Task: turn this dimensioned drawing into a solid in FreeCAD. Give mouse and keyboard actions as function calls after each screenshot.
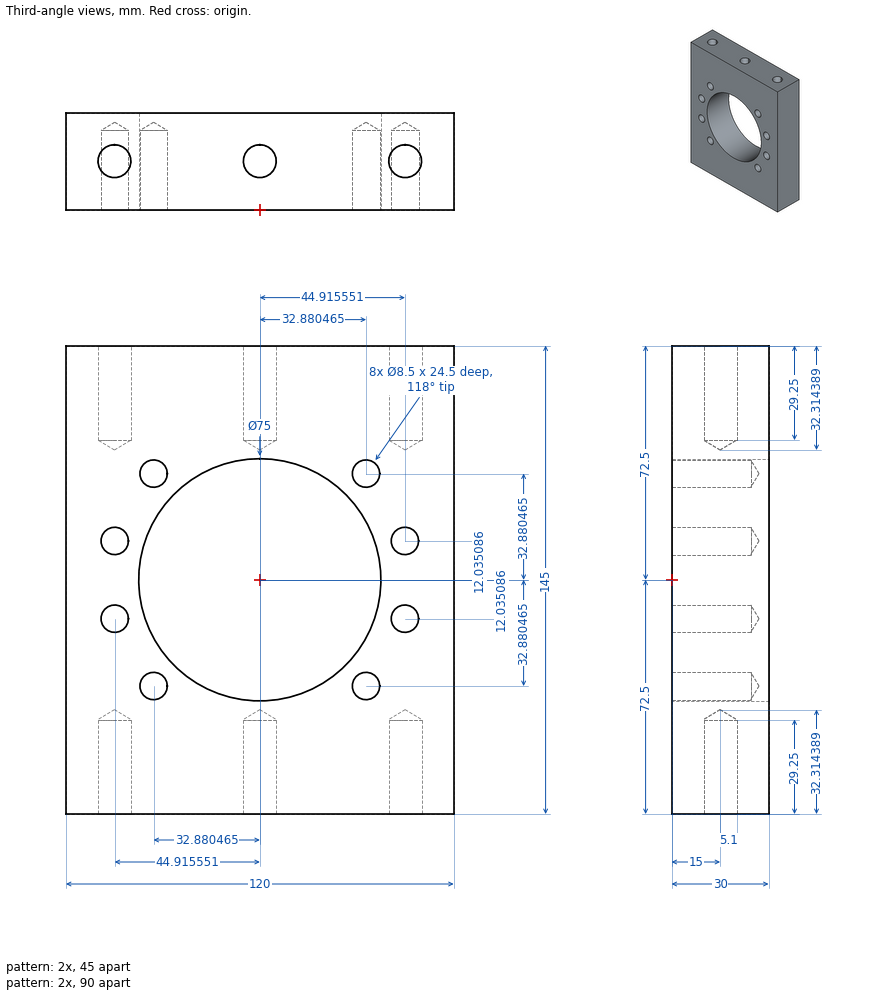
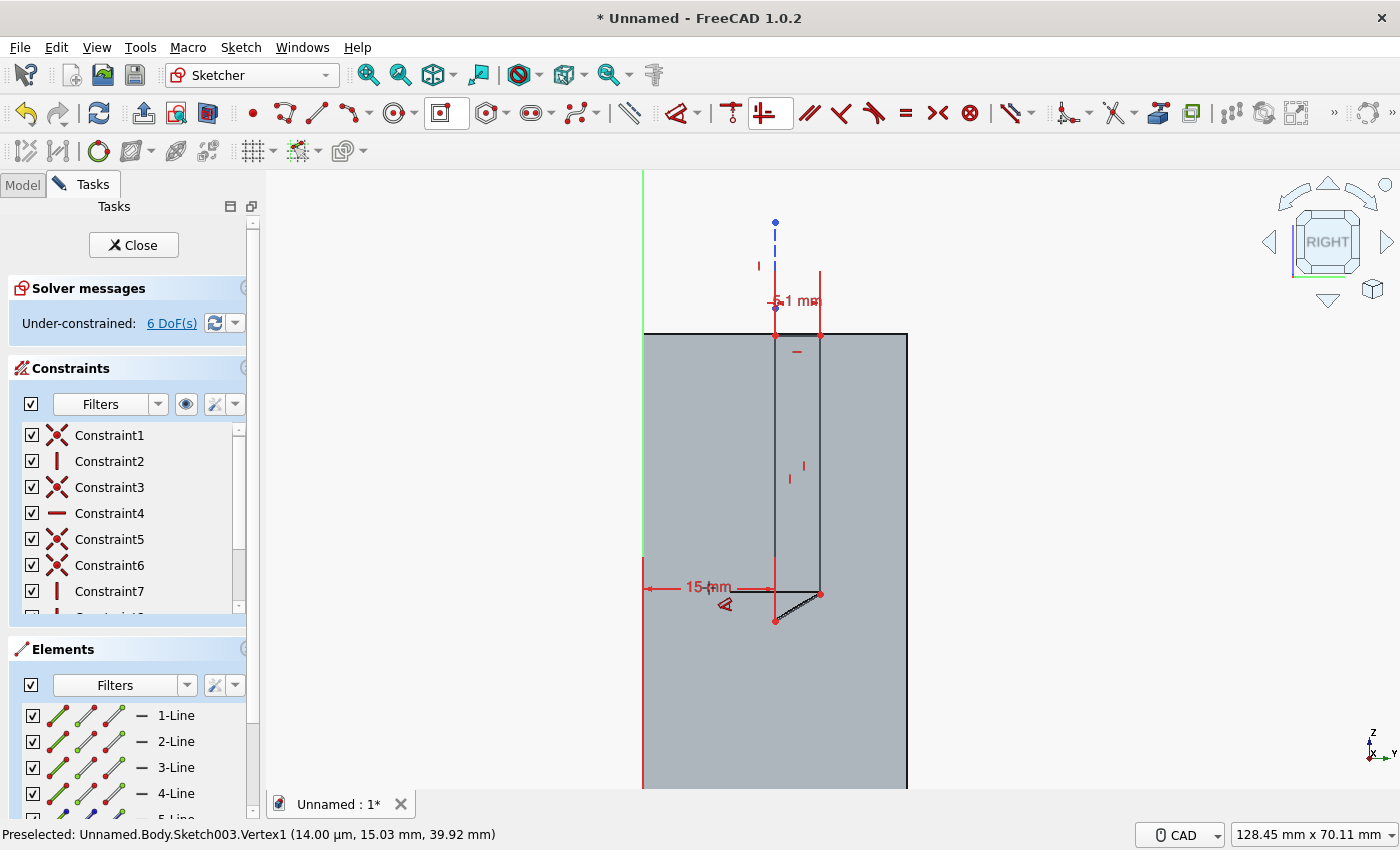
click(775, 308)
click(709, 274)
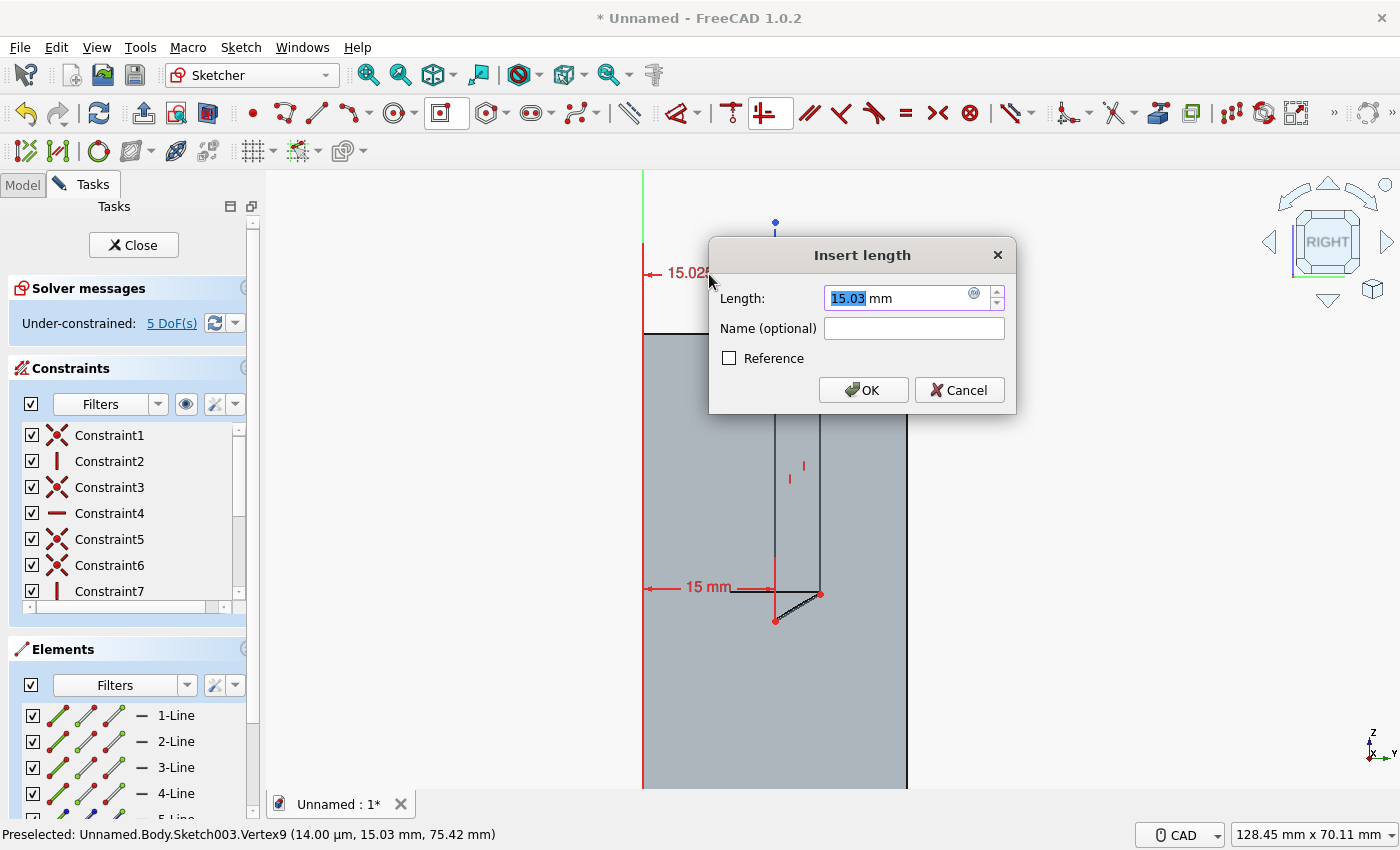
text(15)
key(Return)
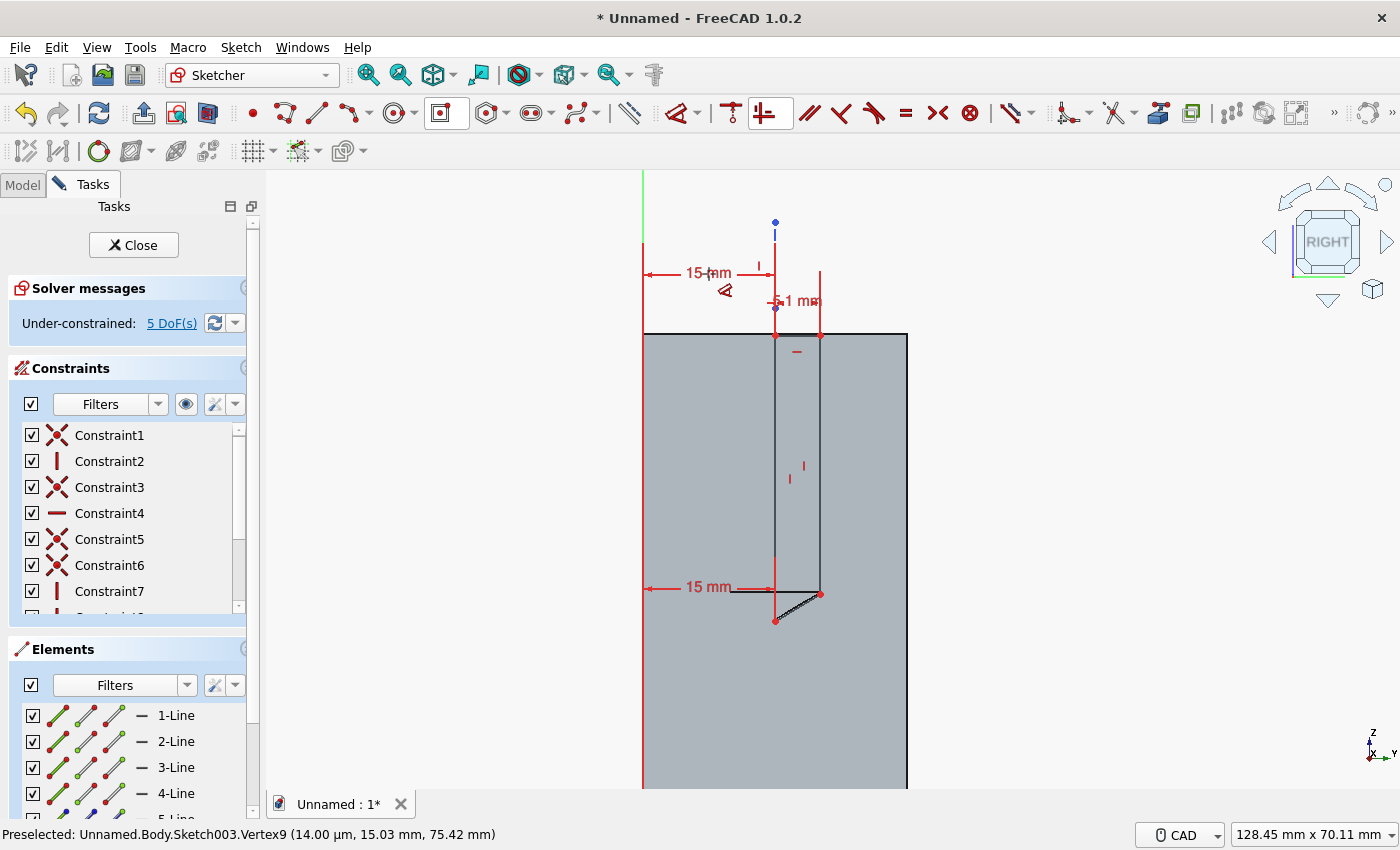
click(820, 517)
click(854, 465)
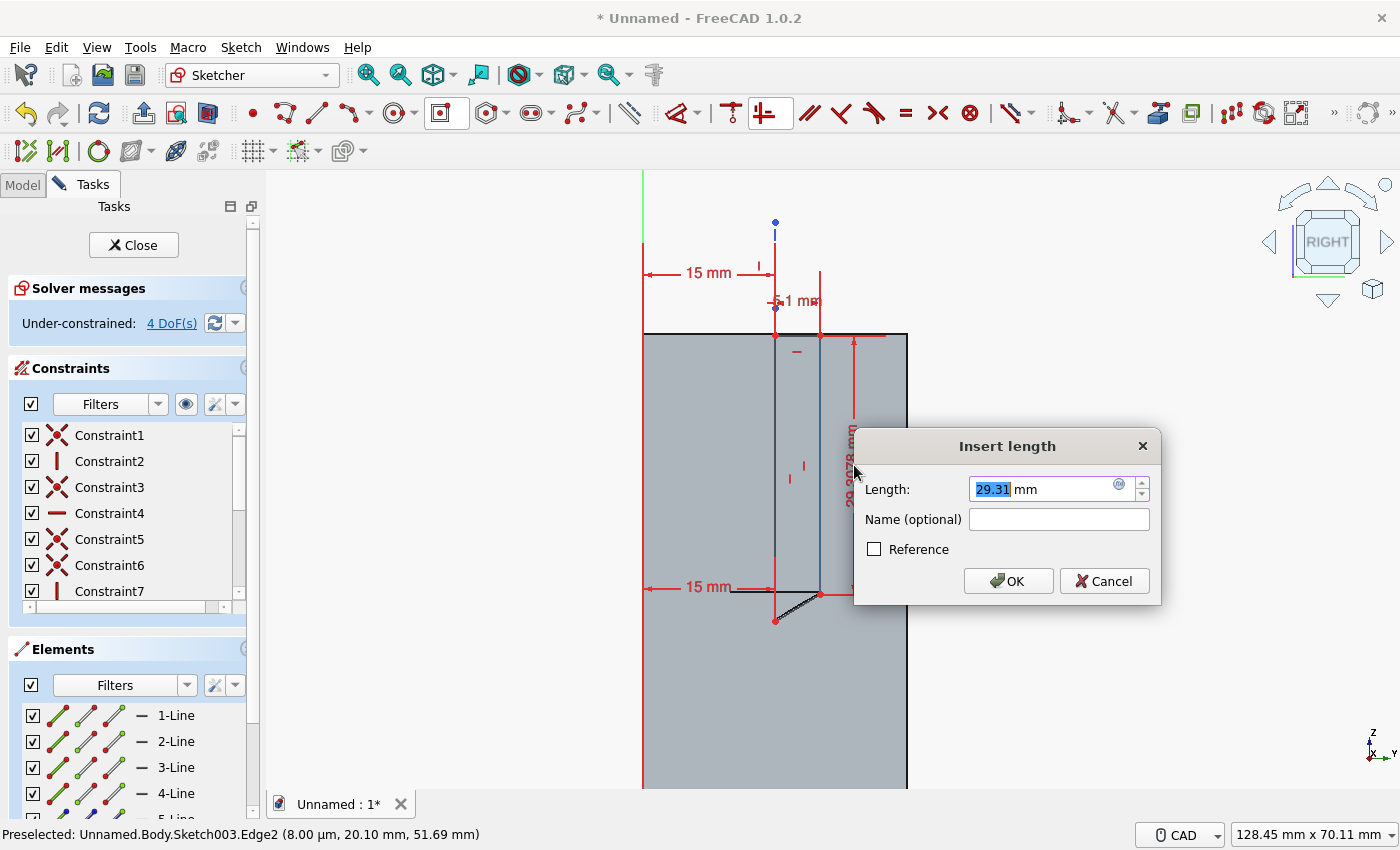
text(29.25)
key(Return)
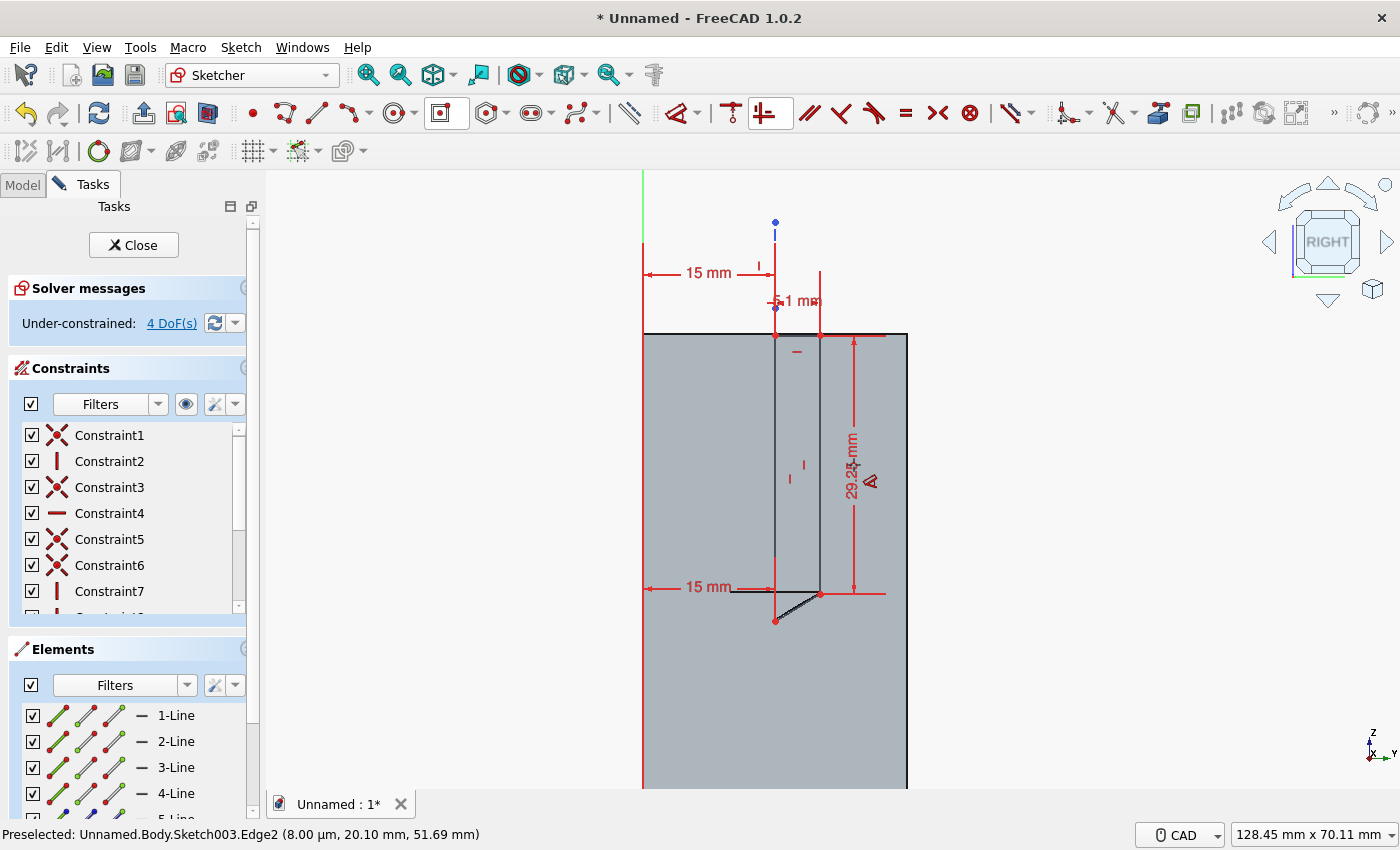
click(820, 336)
click(854, 548)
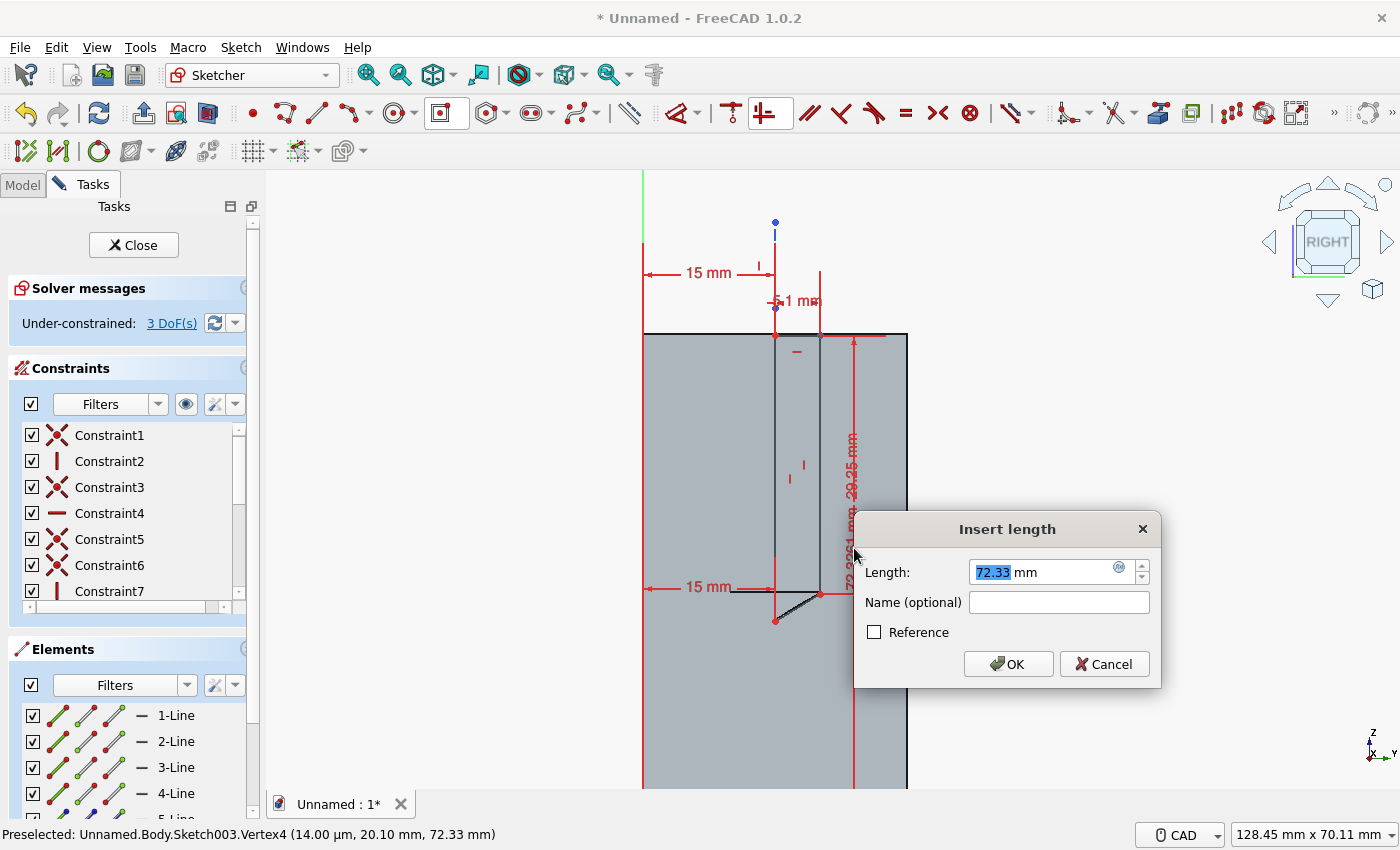
text(72.5)
key(Return)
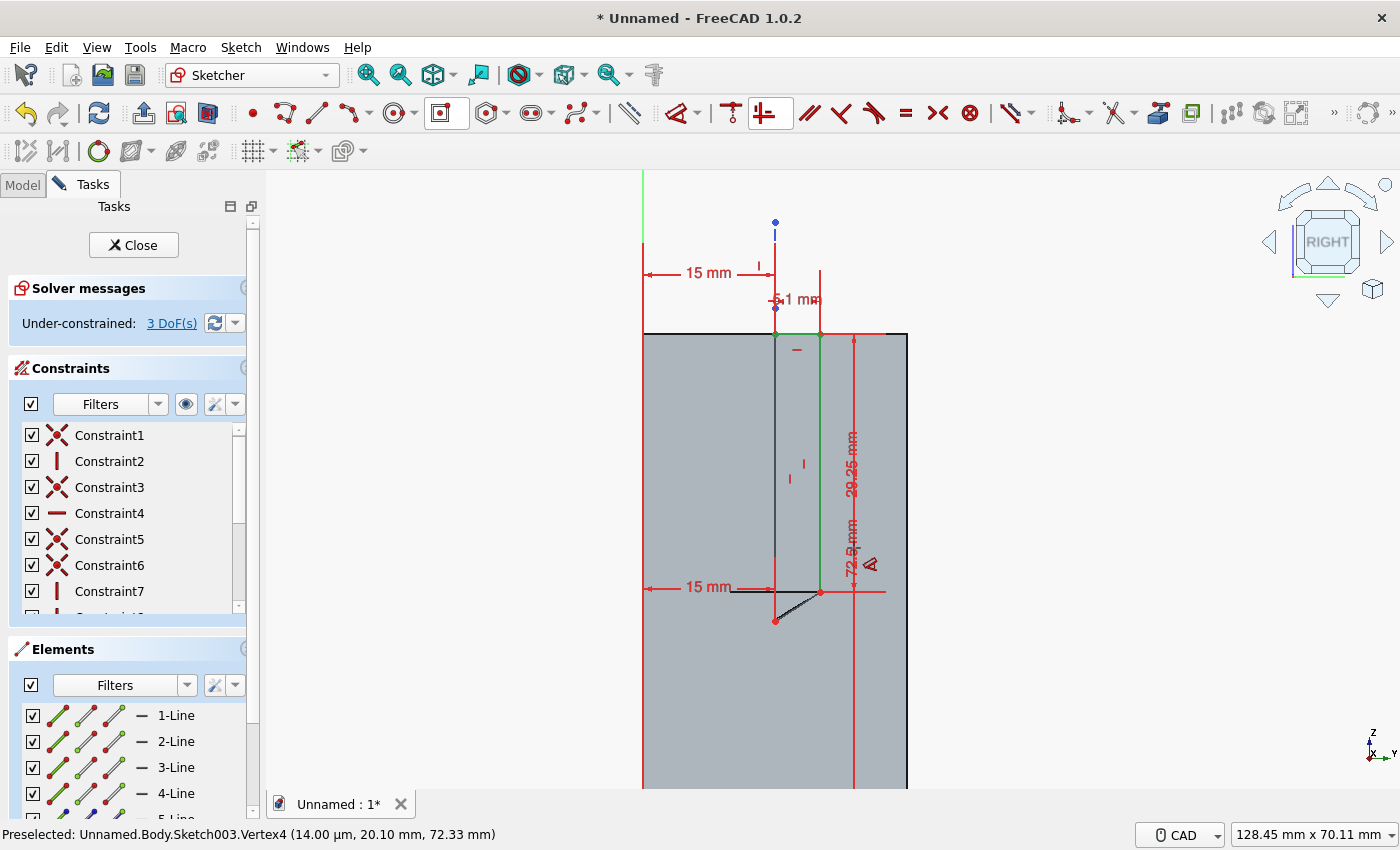
click(775, 421)
click(741, 478)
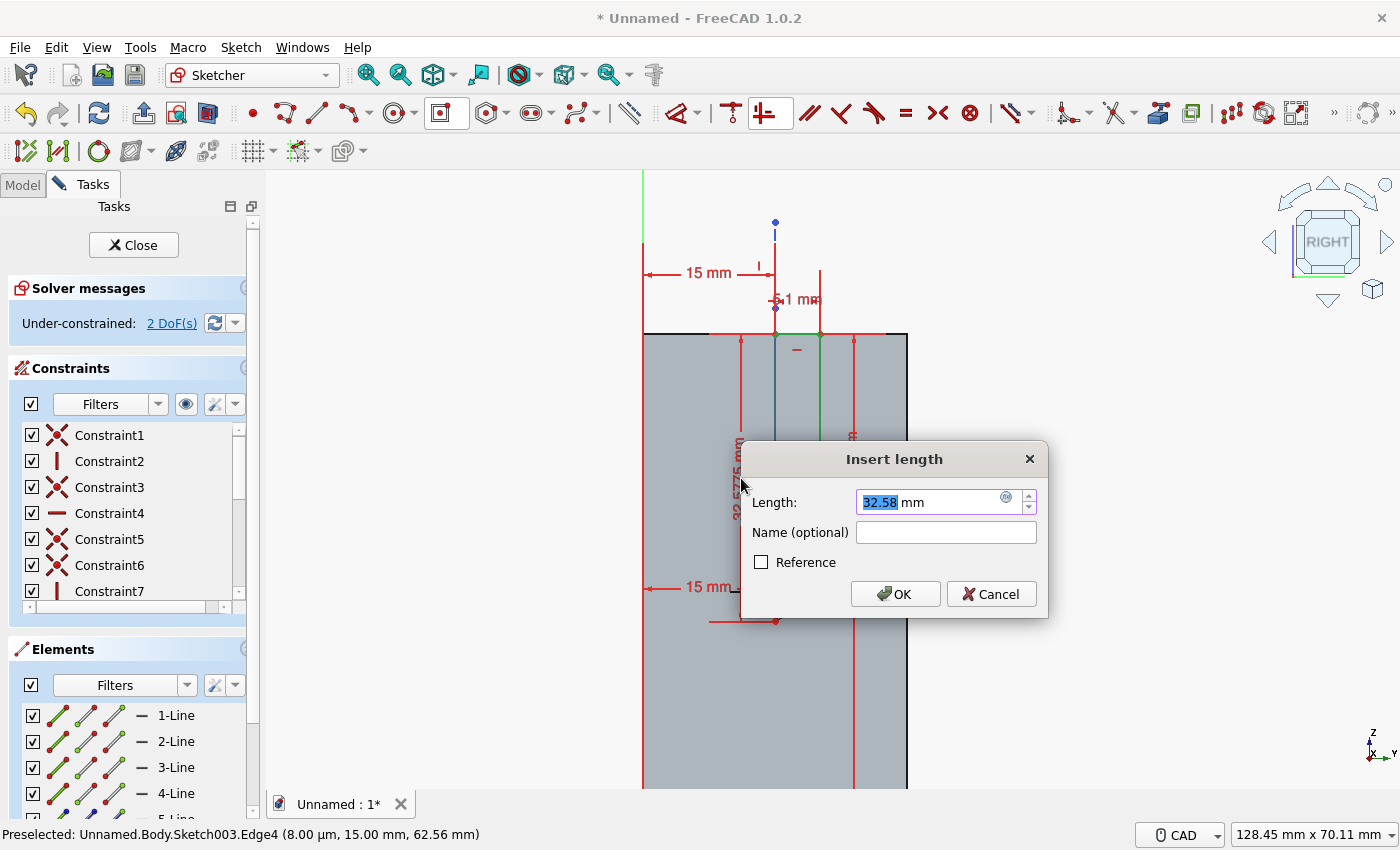
text(32.314389)
key(Return)
key(Escape)